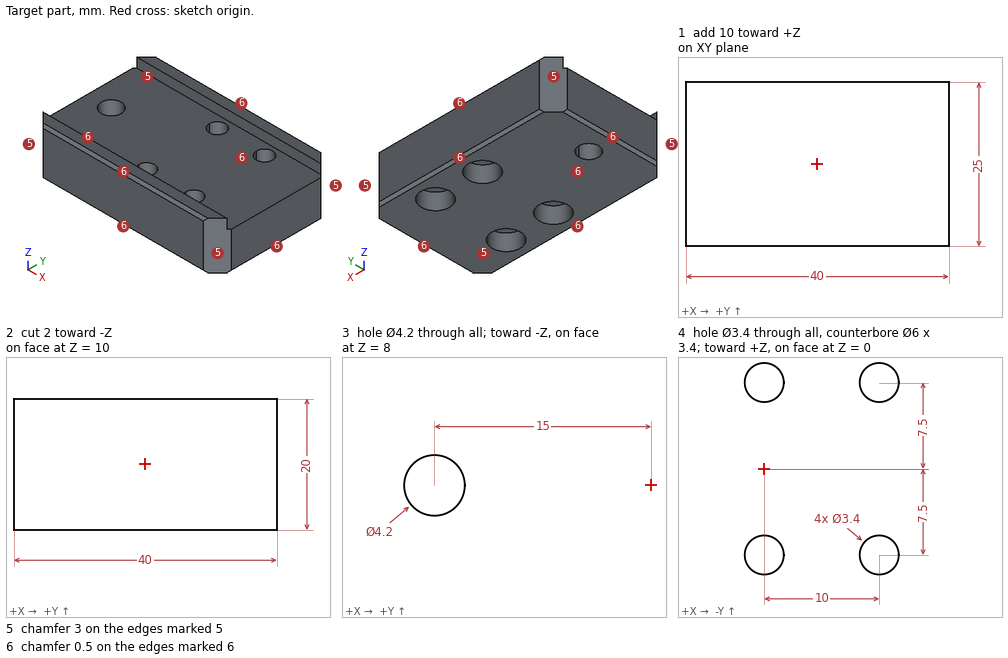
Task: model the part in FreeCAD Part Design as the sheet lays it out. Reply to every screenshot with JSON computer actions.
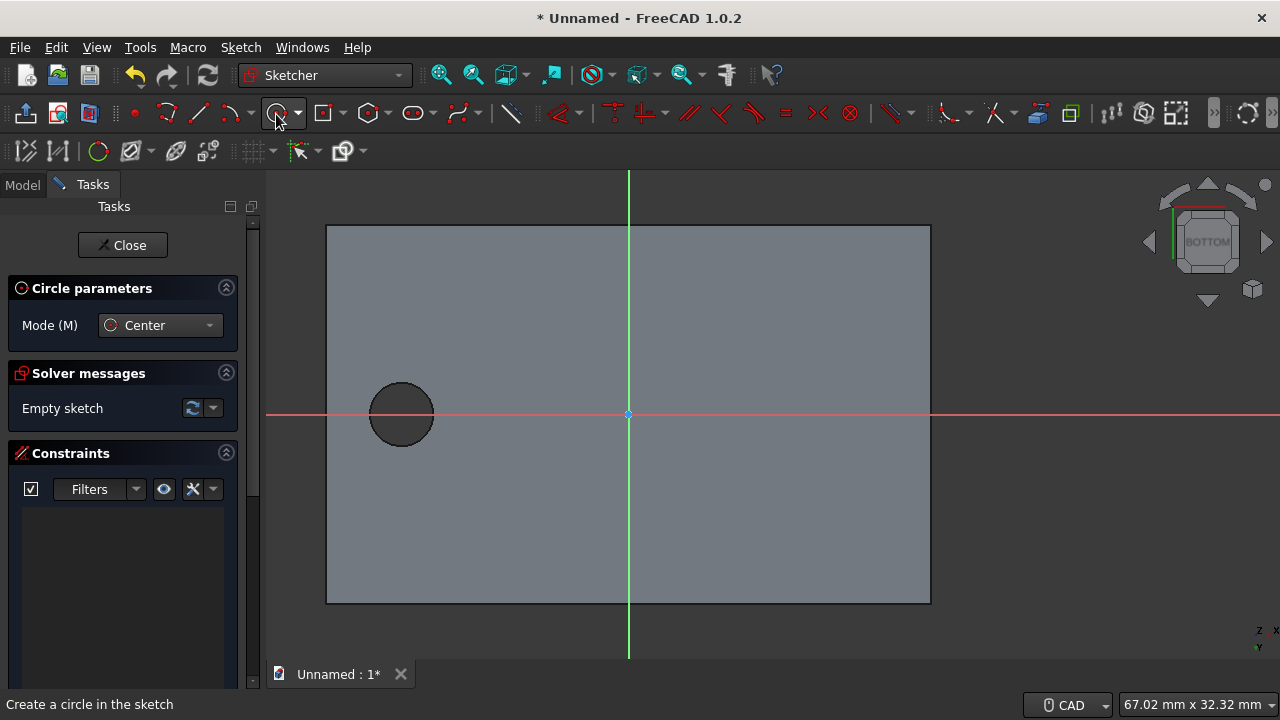
{"action": "left_click", "coordinate": [780, 528]}
{"action": "left_click", "coordinate": [798, 510]}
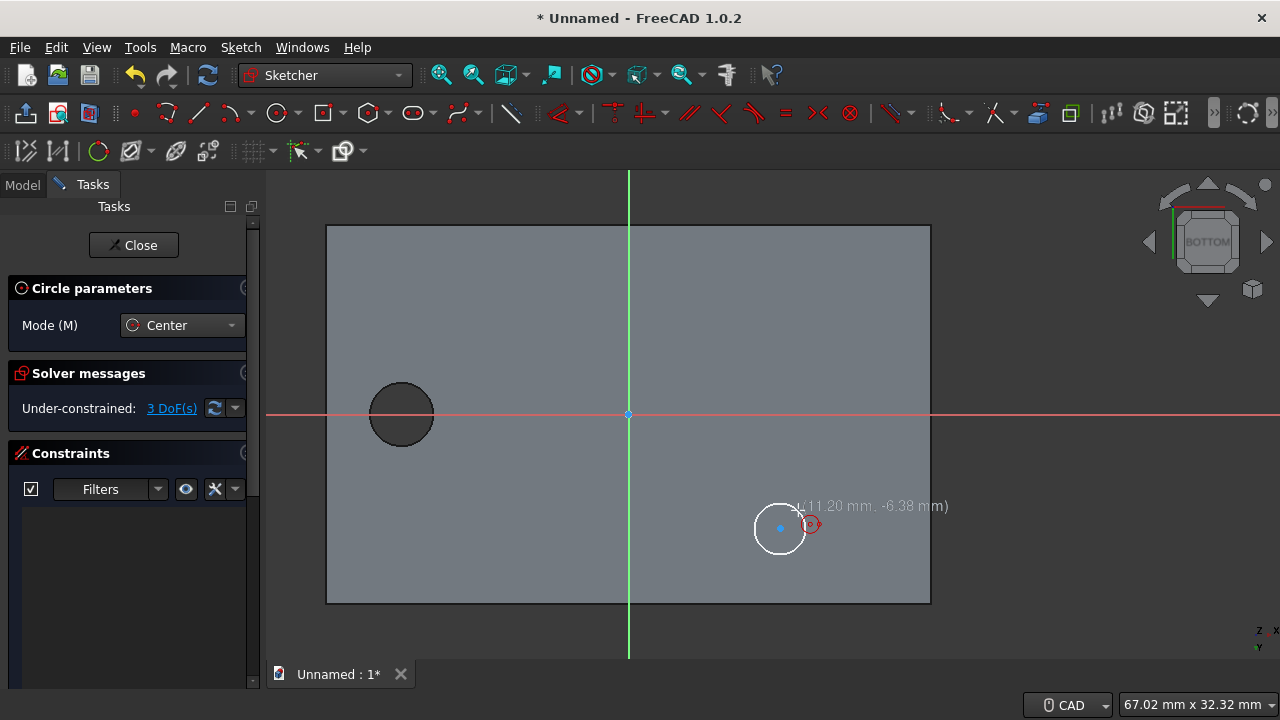
{"action": "left_click", "coordinate": [780, 301]}
{"action": "left_click", "coordinate": [798, 283]}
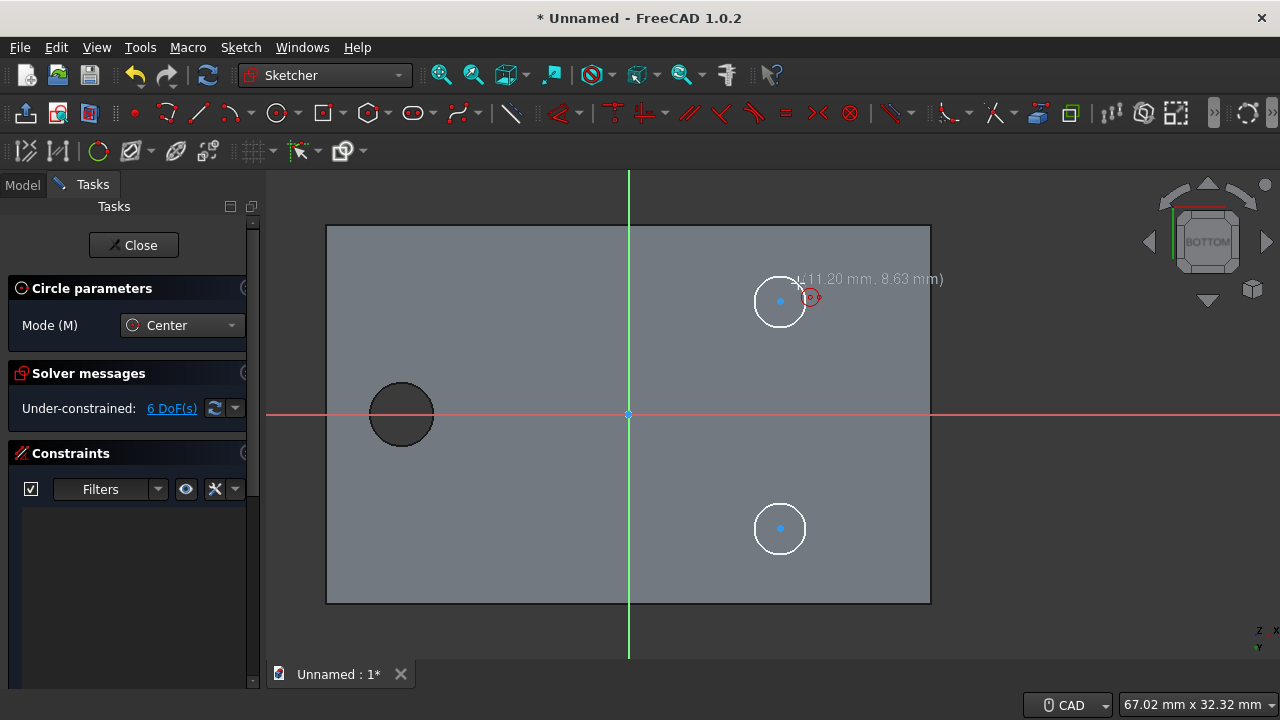
{"action": "left_click", "coordinate": [629, 528]}
{"action": "left_click", "coordinate": [647, 510]}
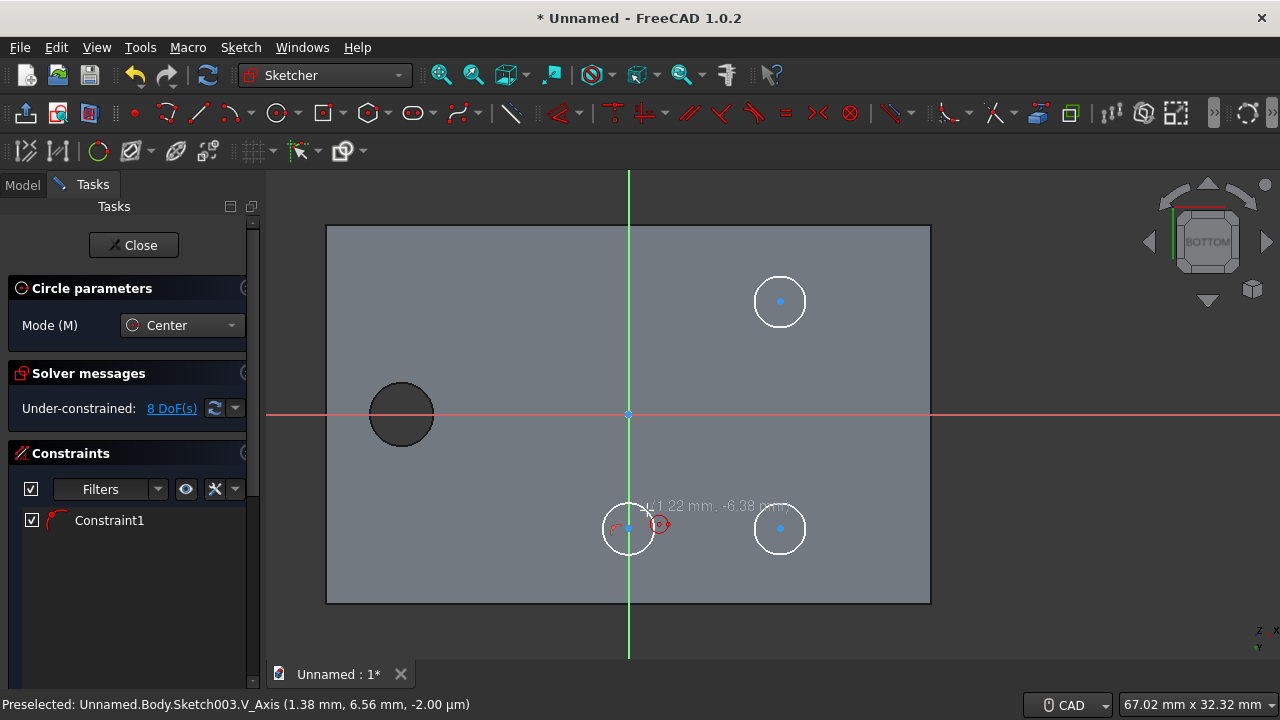
{"action": "left_click", "coordinate": [629, 301]}
{"action": "left_click", "coordinate": [647, 283]}
{"action": "key", "text": "Escape"}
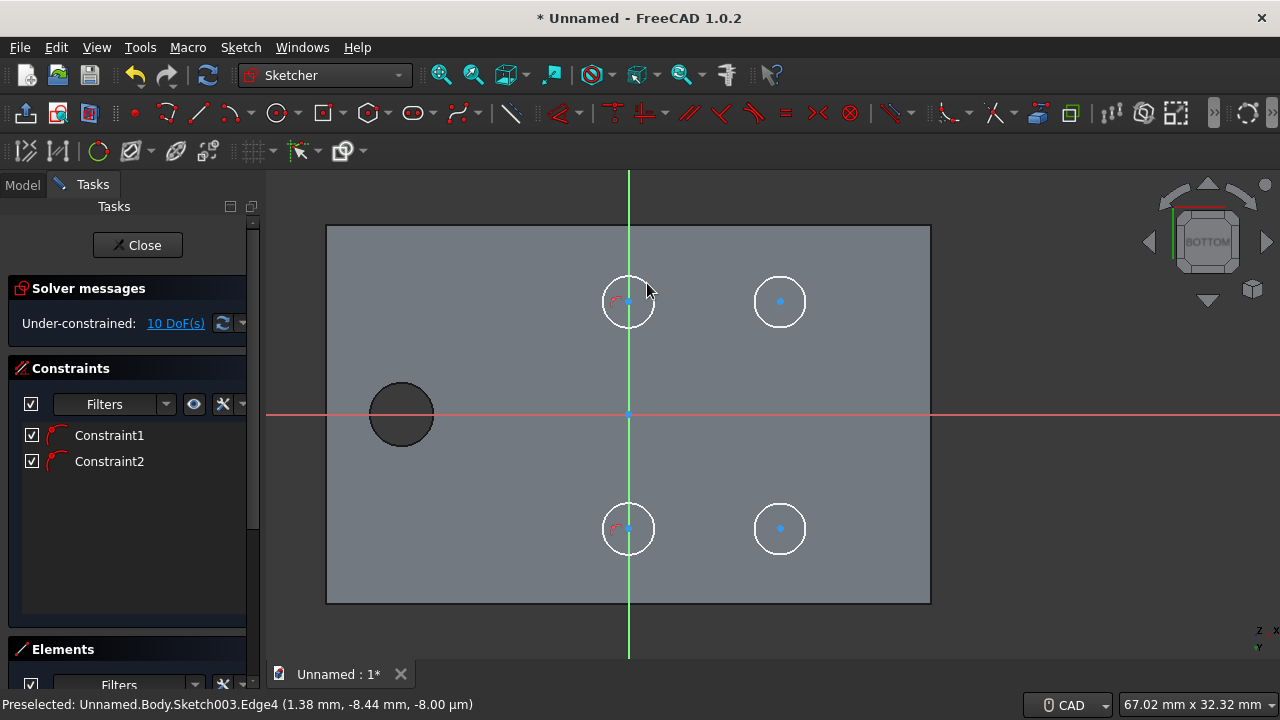
{"action": "left_click", "coordinate": [798, 511]}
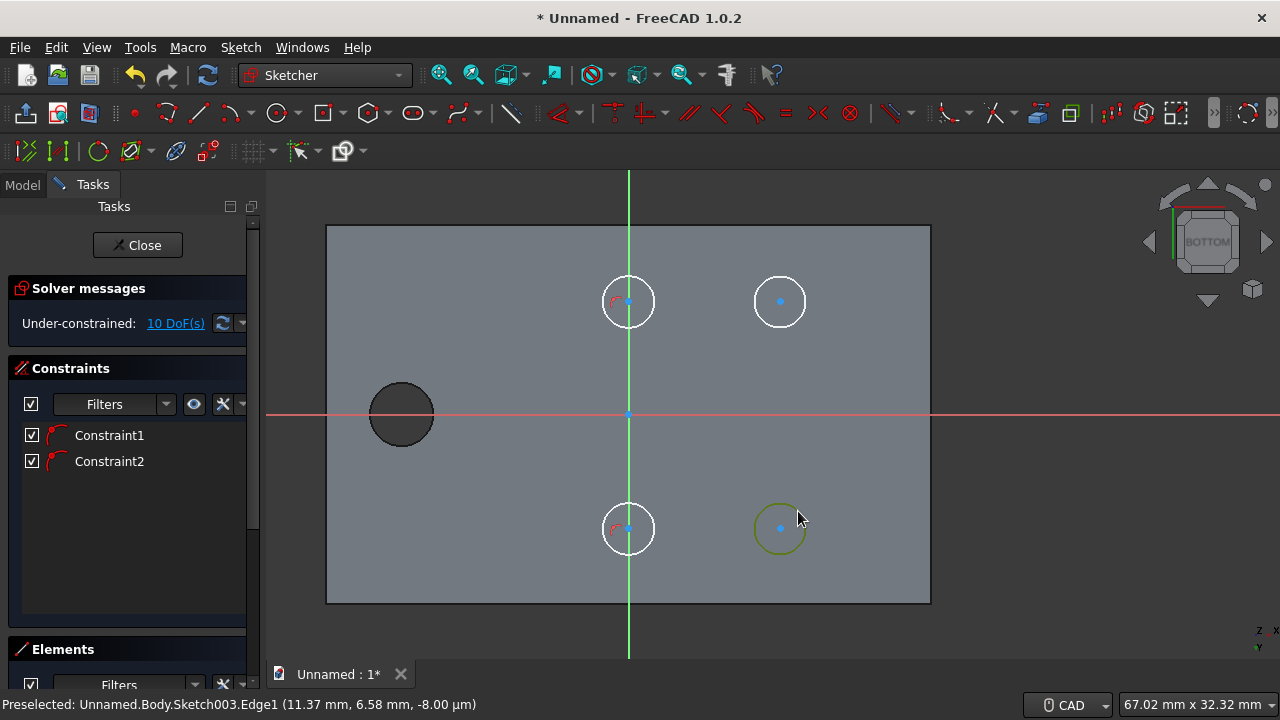
{"action": "left_click", "coordinate": [798, 284]}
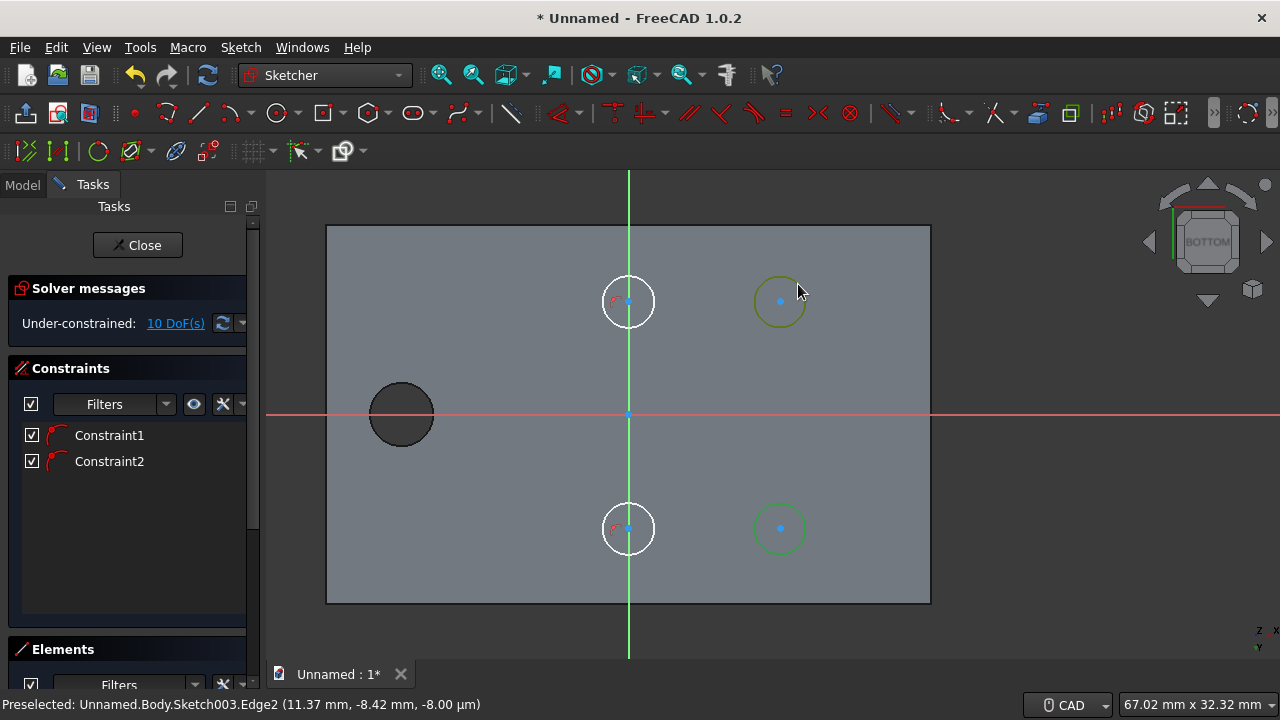
{"action": "left_click", "coordinate": [647, 511]}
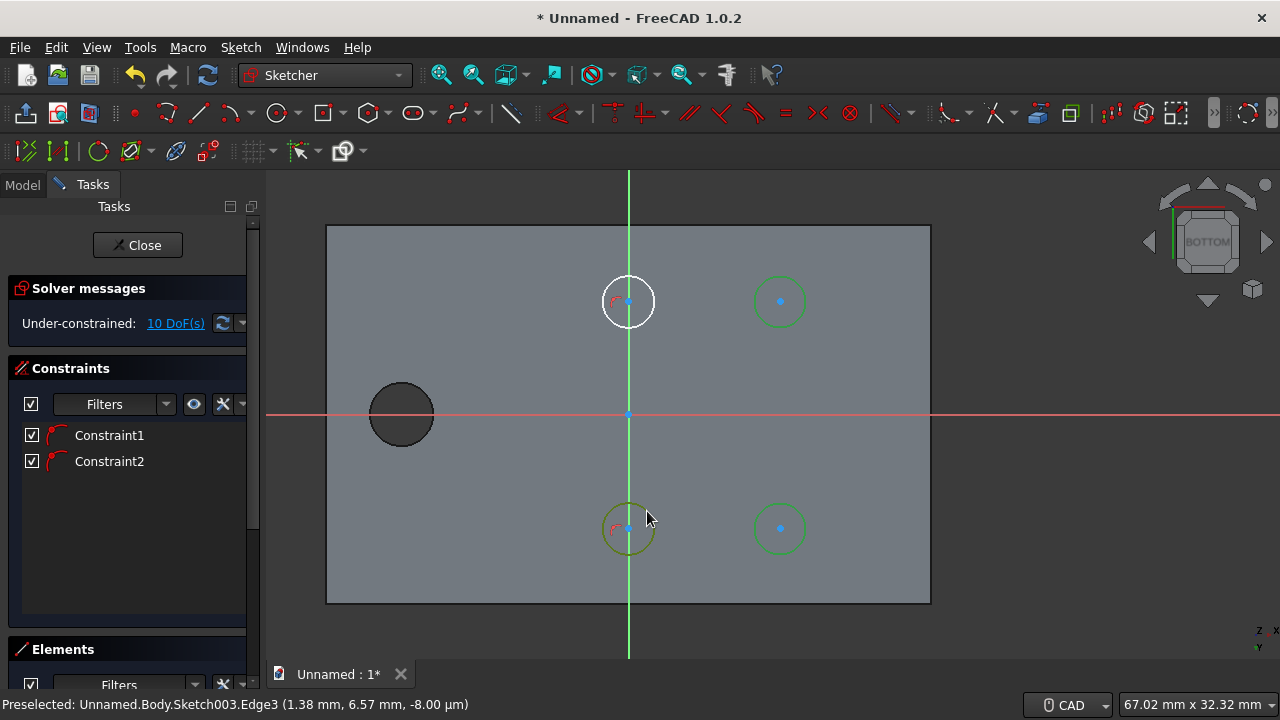
{"action": "left_click", "coordinate": [647, 284]}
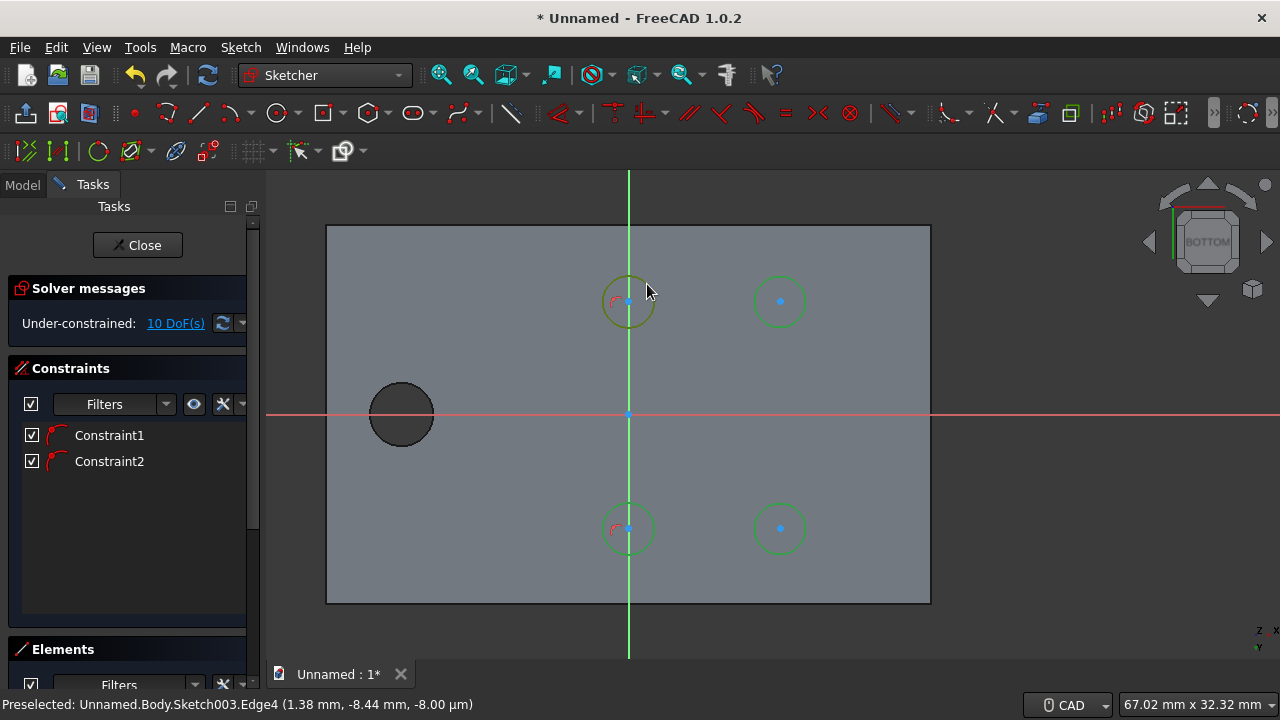
{"action": "left_click", "coordinate": [786, 114]}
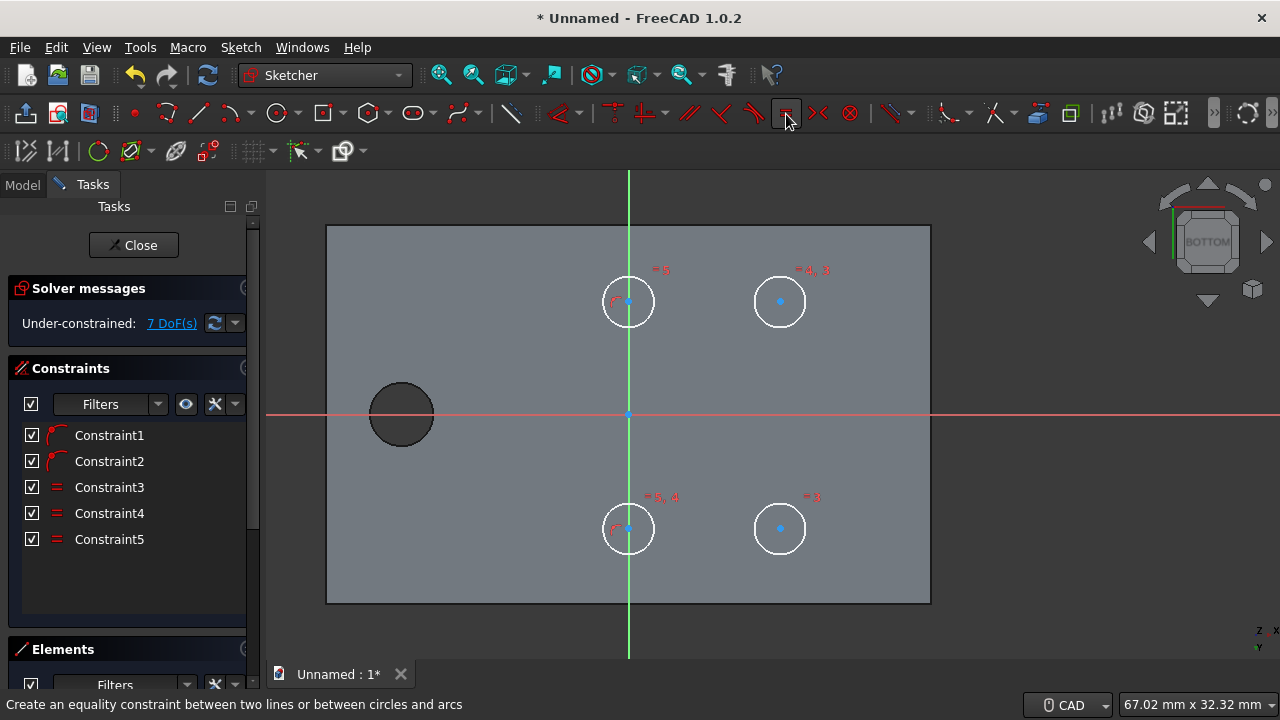
{"action": "left_click", "coordinate": [780, 529]}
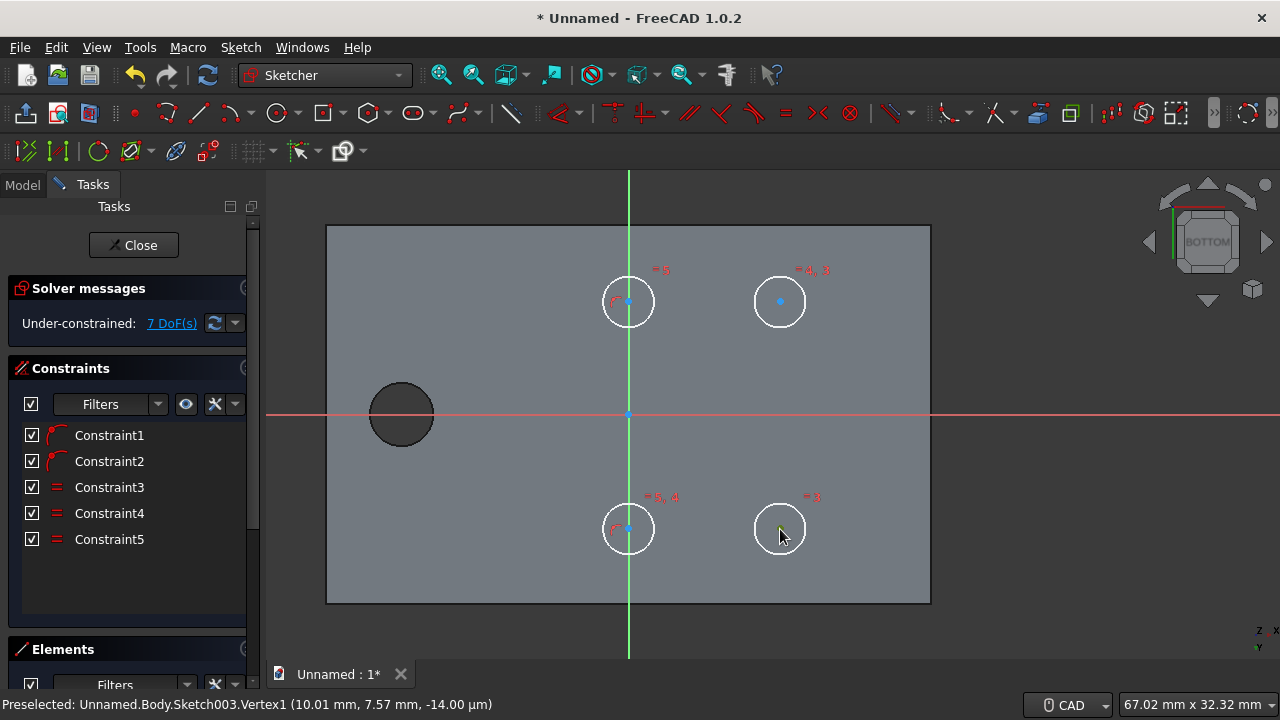
{"action": "left_click", "coordinate": [780, 302]}